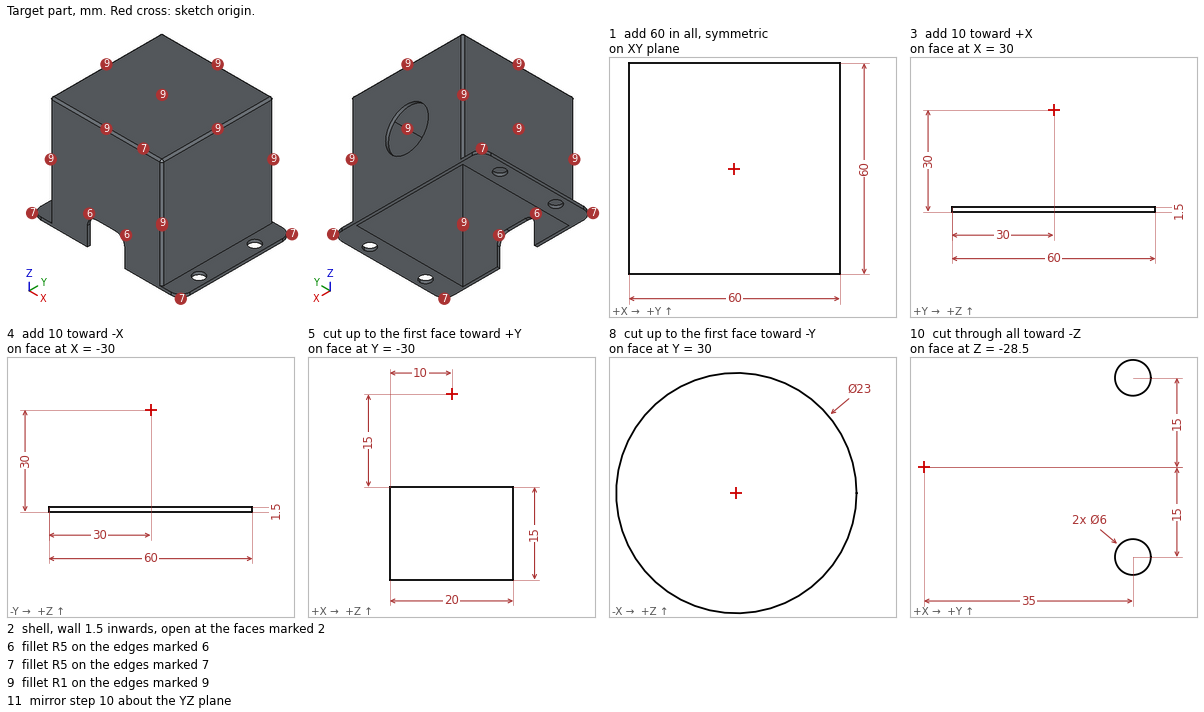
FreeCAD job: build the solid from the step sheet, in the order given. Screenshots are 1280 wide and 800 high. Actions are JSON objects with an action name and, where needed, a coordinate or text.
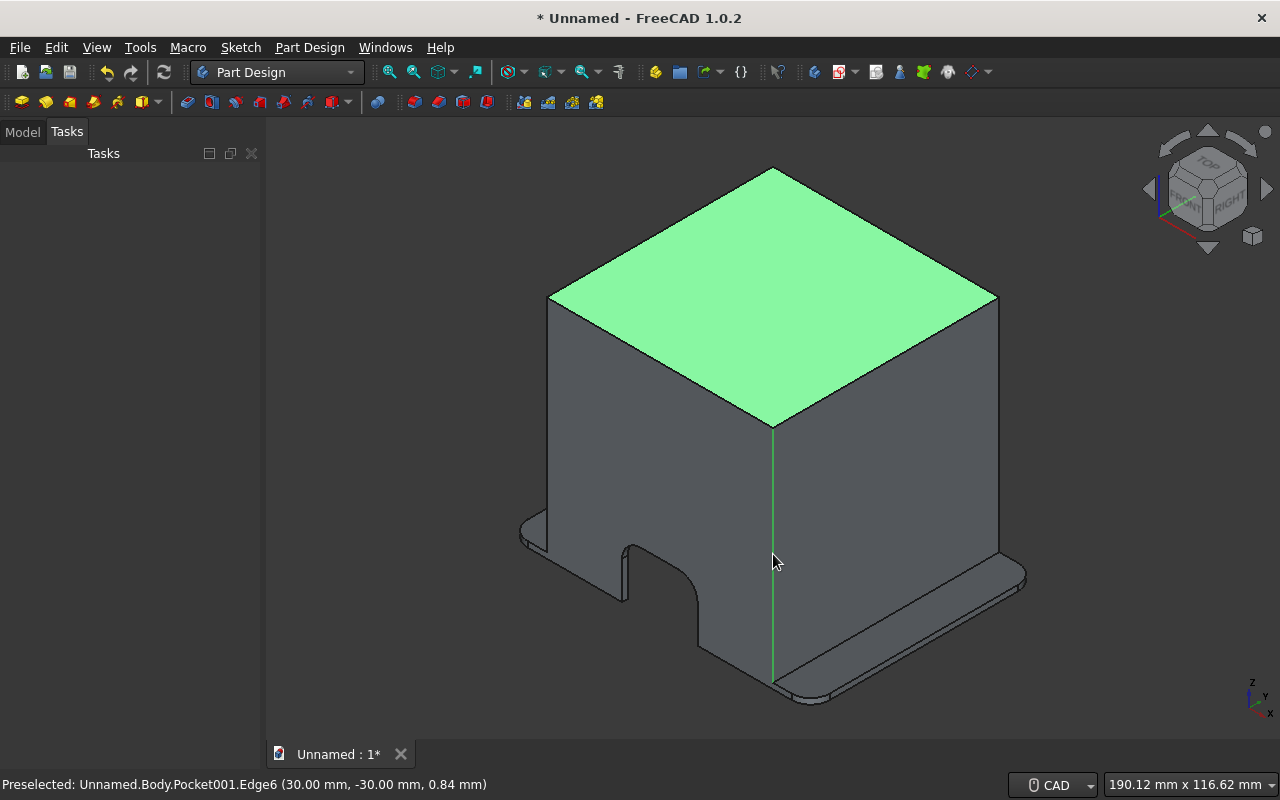
{"action": "key", "text": "2"}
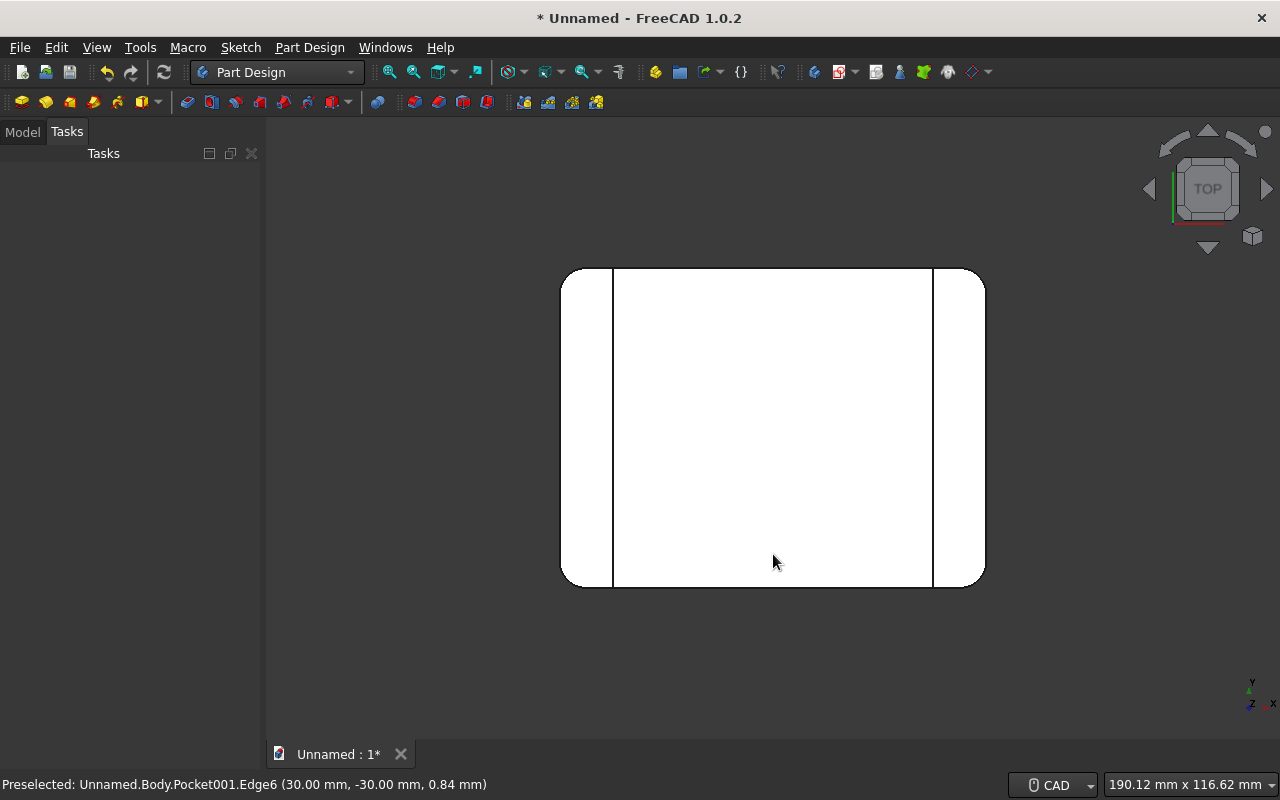
{"action": "key", "text": "1"}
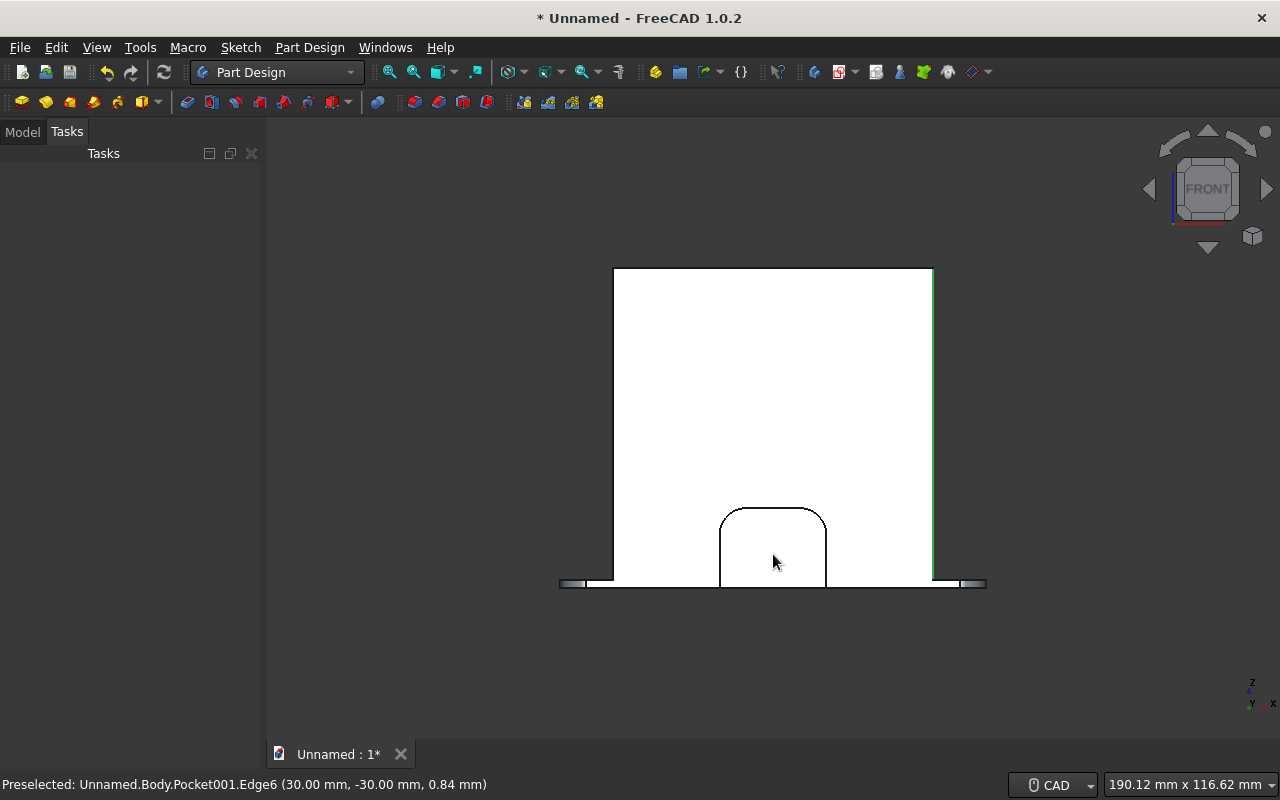
{"action": "left_click", "coordinate": [613, 423], "text": "ctrl"}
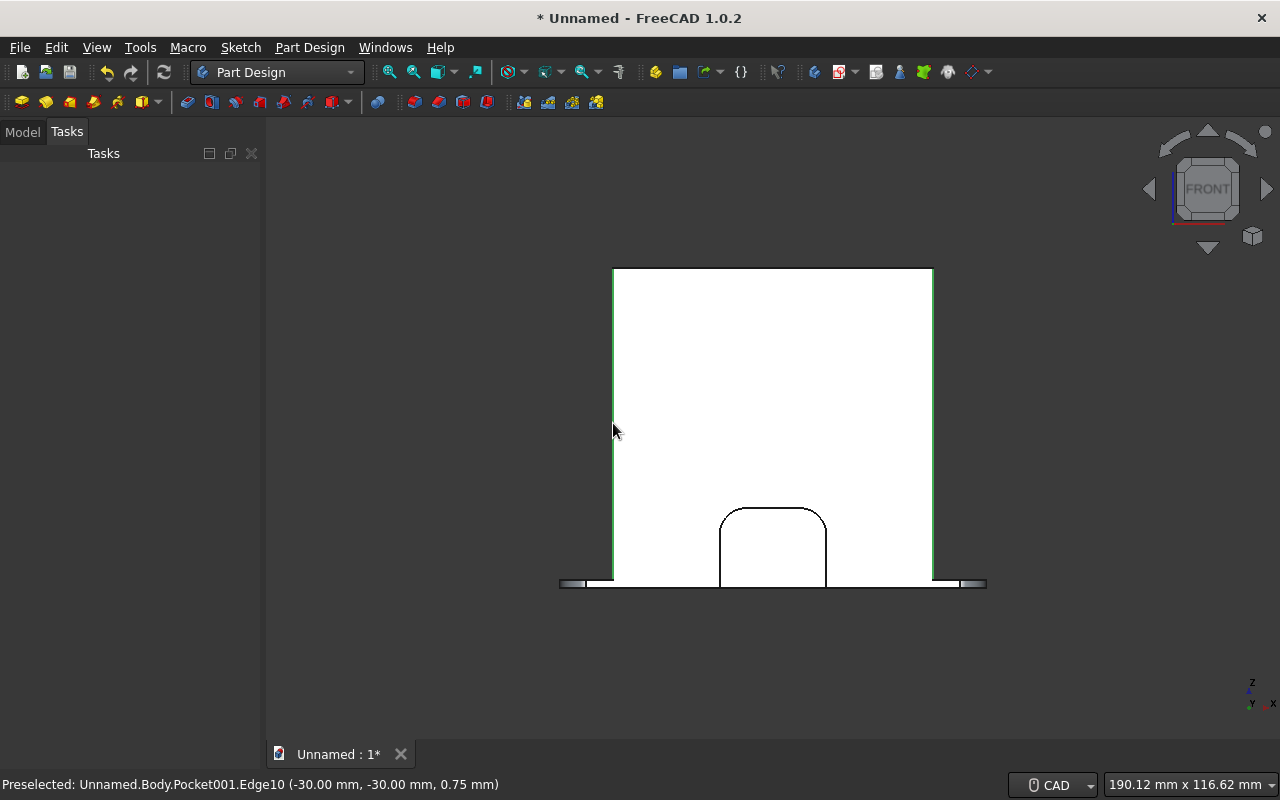
{"action": "key", "text": "3"}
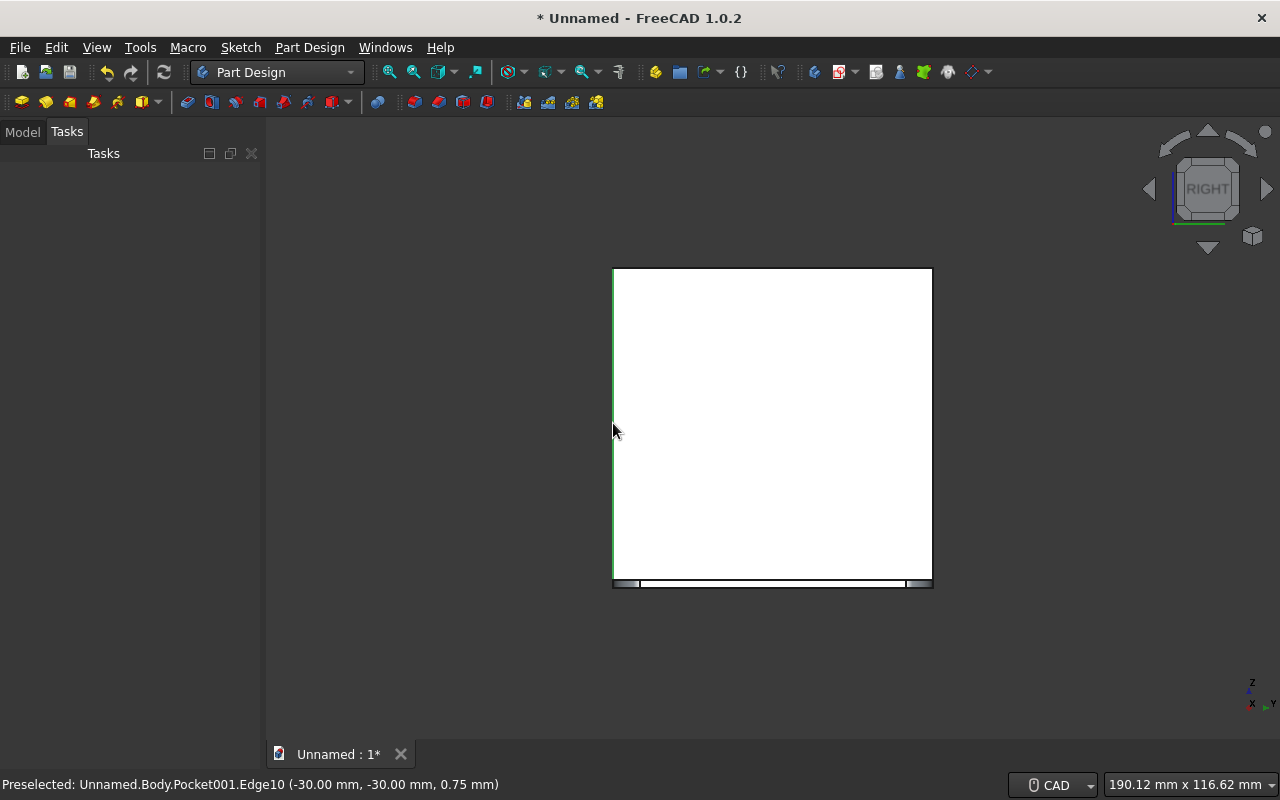
{"action": "left_click", "coordinate": [933, 423], "text": "ctrl"}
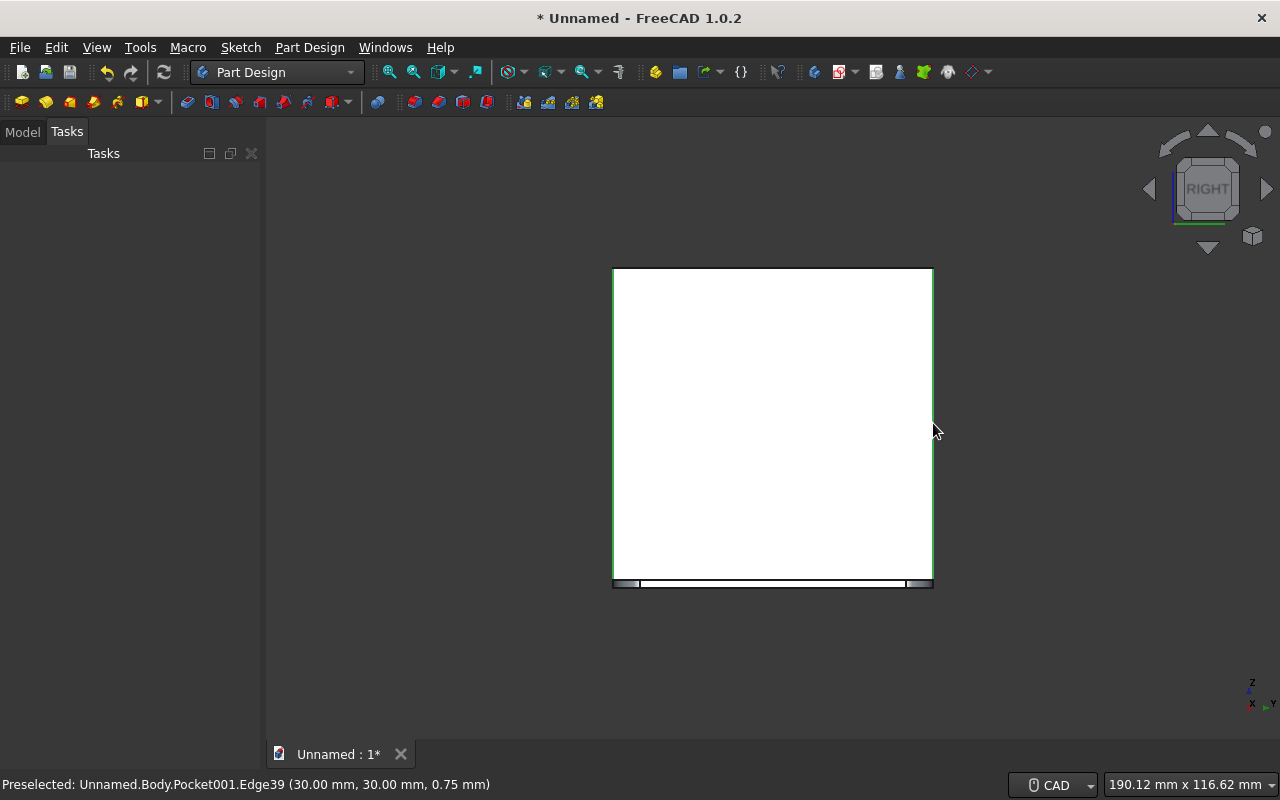
{"action": "left_click", "coordinate": [416, 102]}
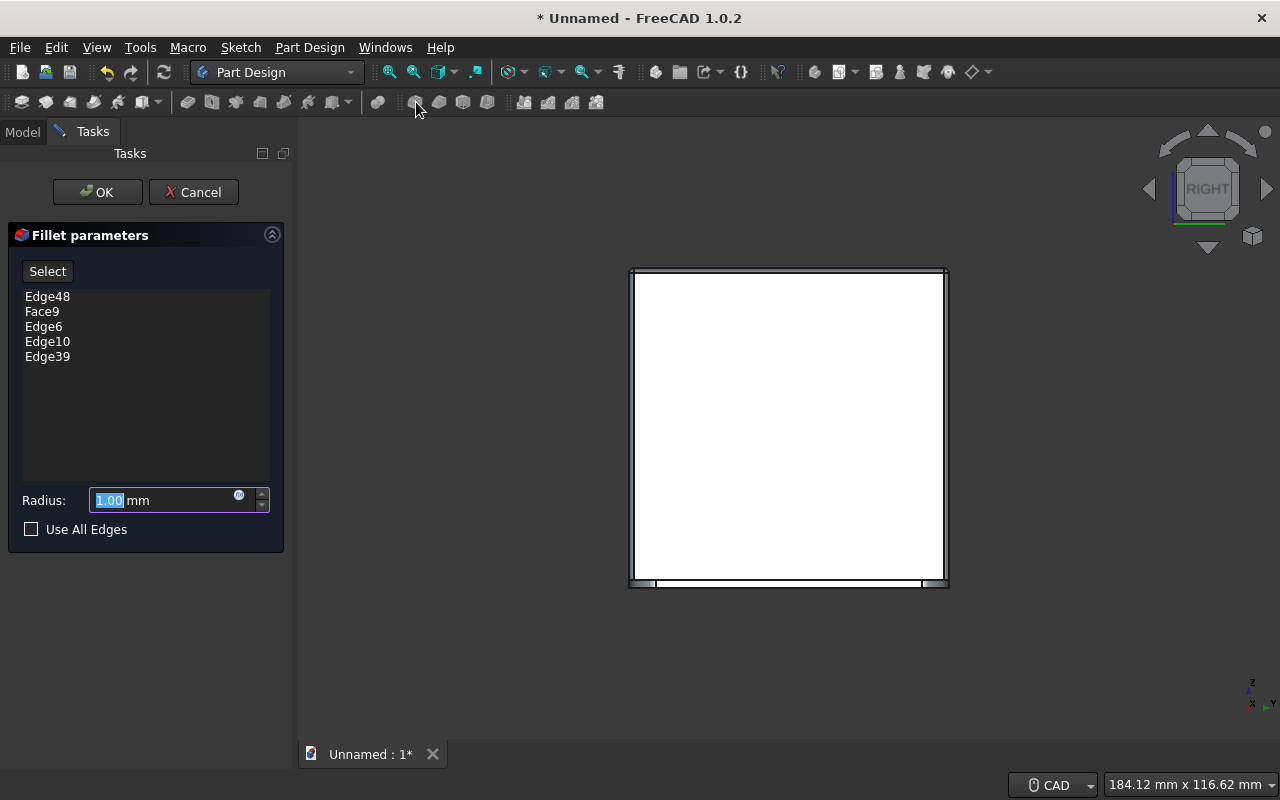
{"action": "type", "text": "1"}
{"action": "key", "text": "Tab"}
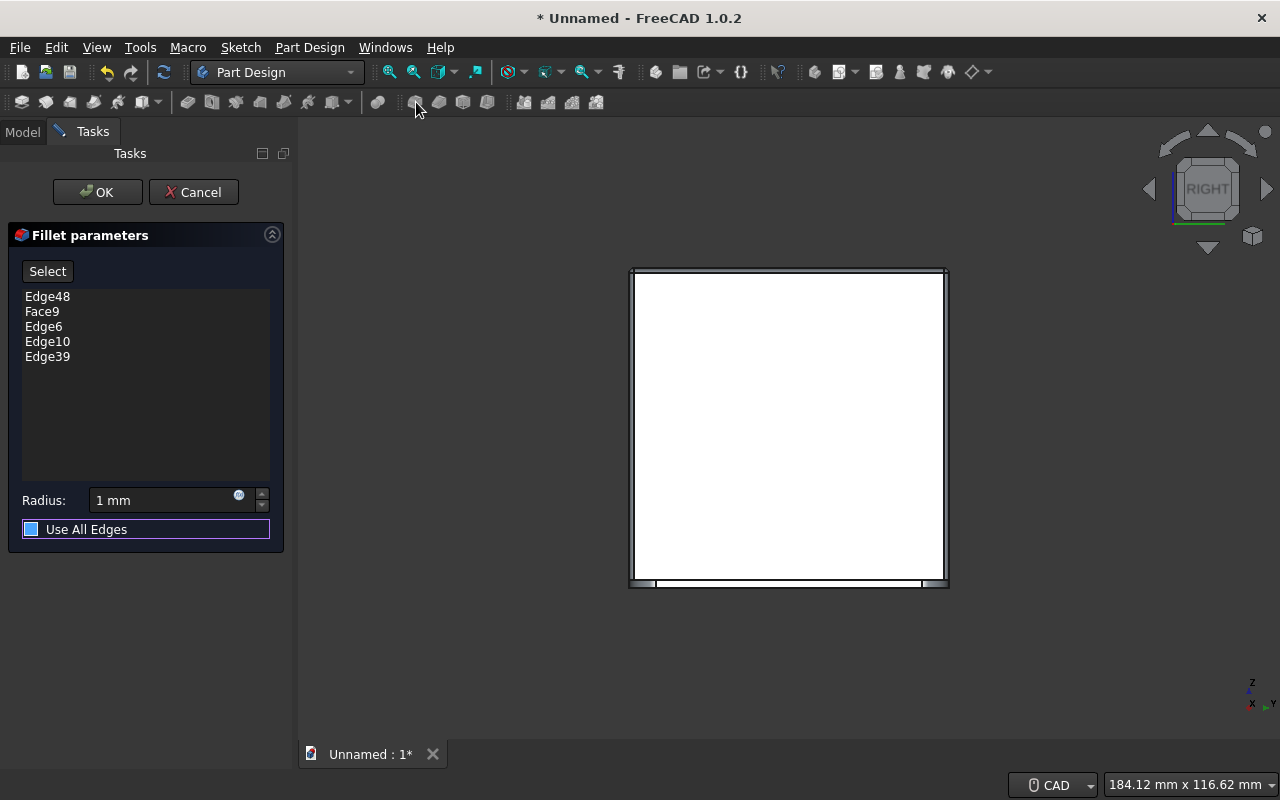
{"action": "left_click", "coordinate": [98, 192]}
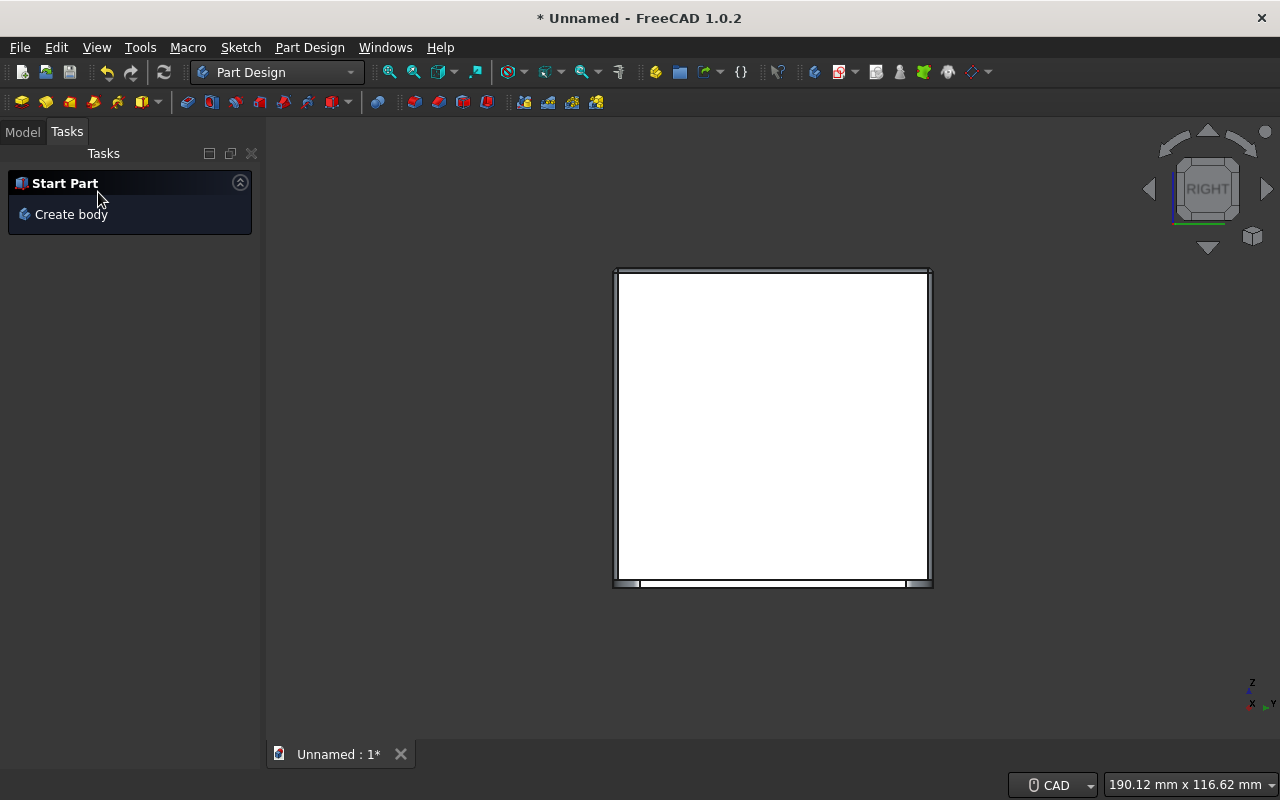
{"action": "key", "text": "0"}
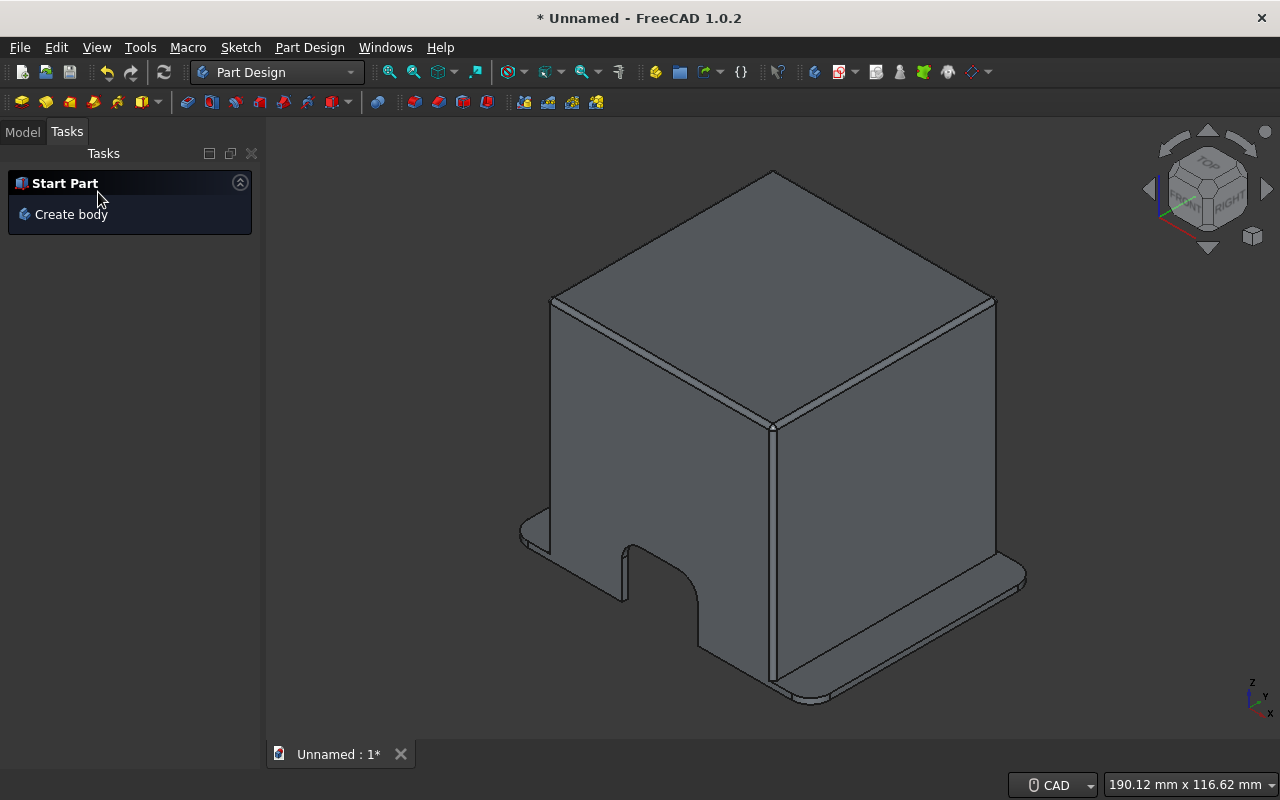
{"action": "left_click", "coordinate": [968, 589]}